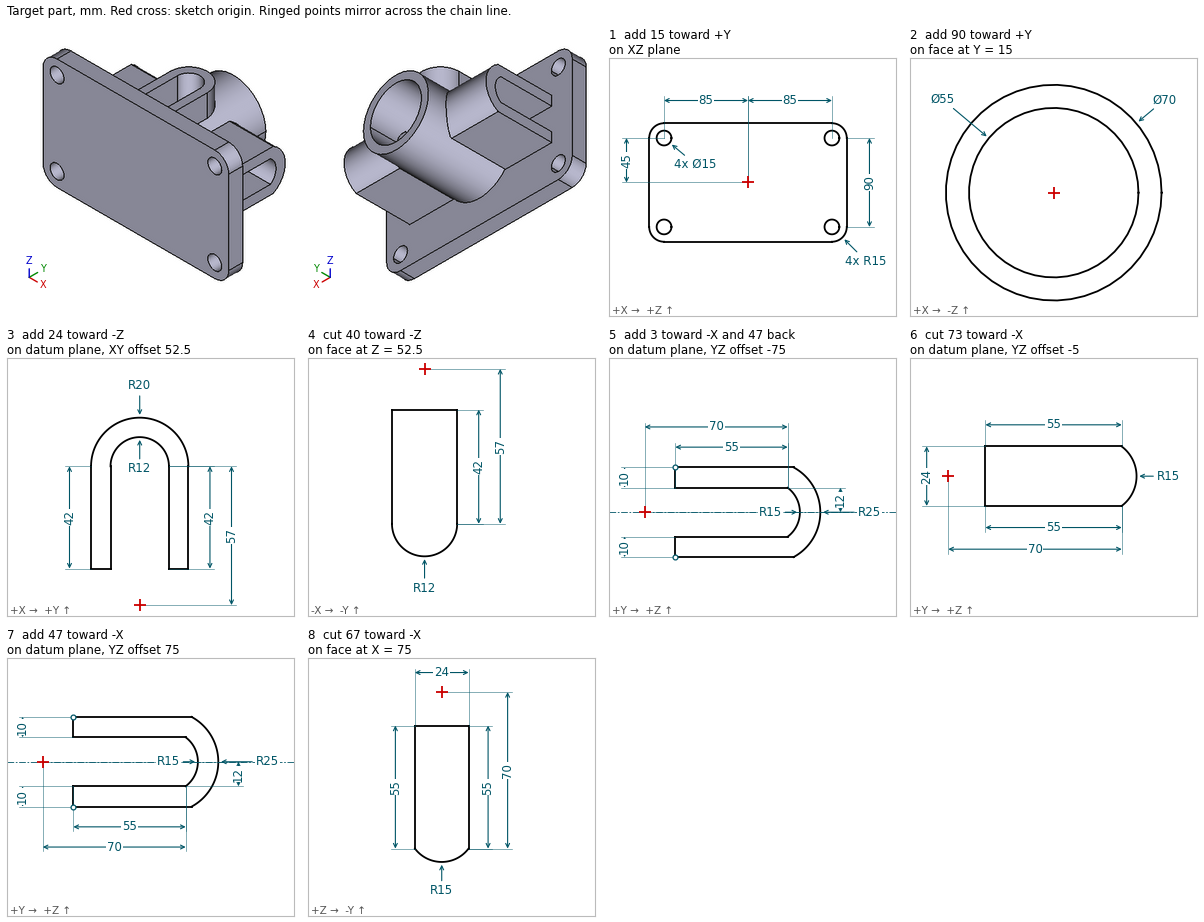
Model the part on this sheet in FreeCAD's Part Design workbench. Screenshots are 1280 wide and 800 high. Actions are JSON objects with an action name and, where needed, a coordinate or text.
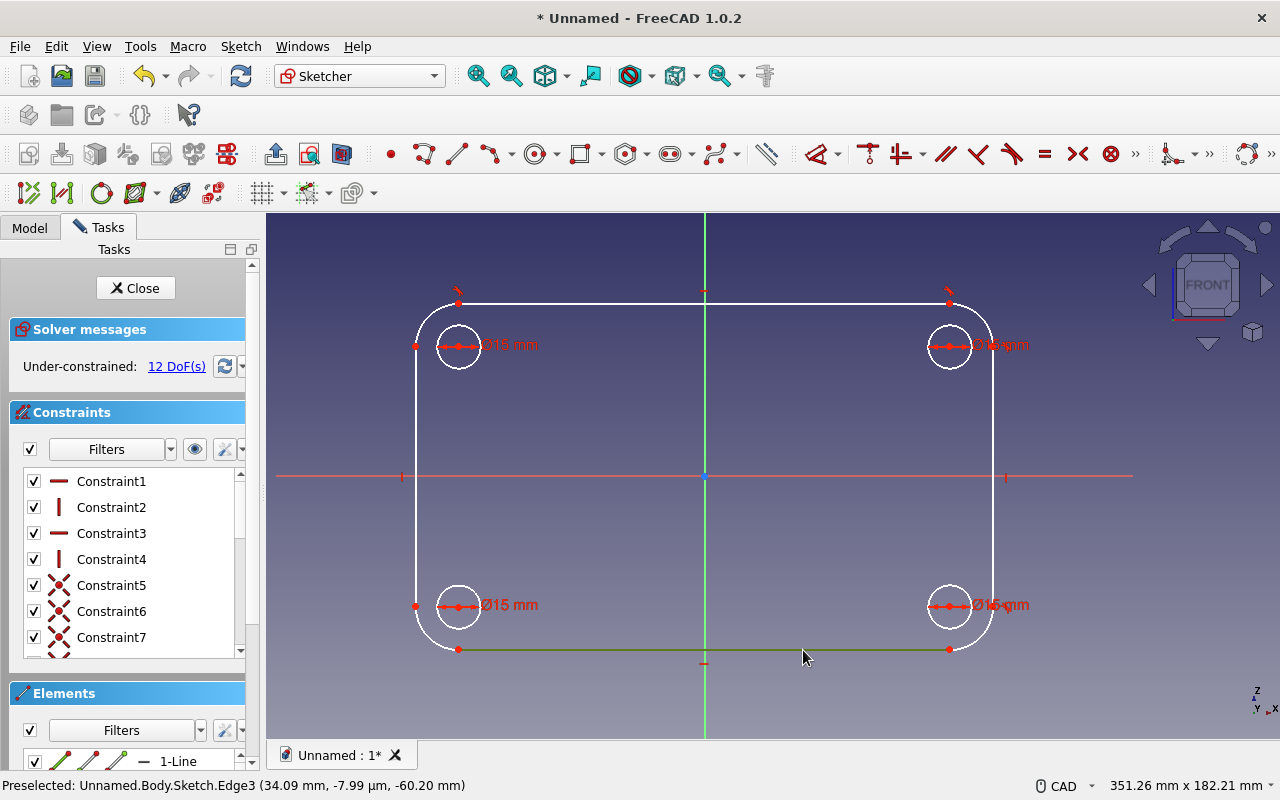
{"action": "left_click", "coordinate": [970, 645]}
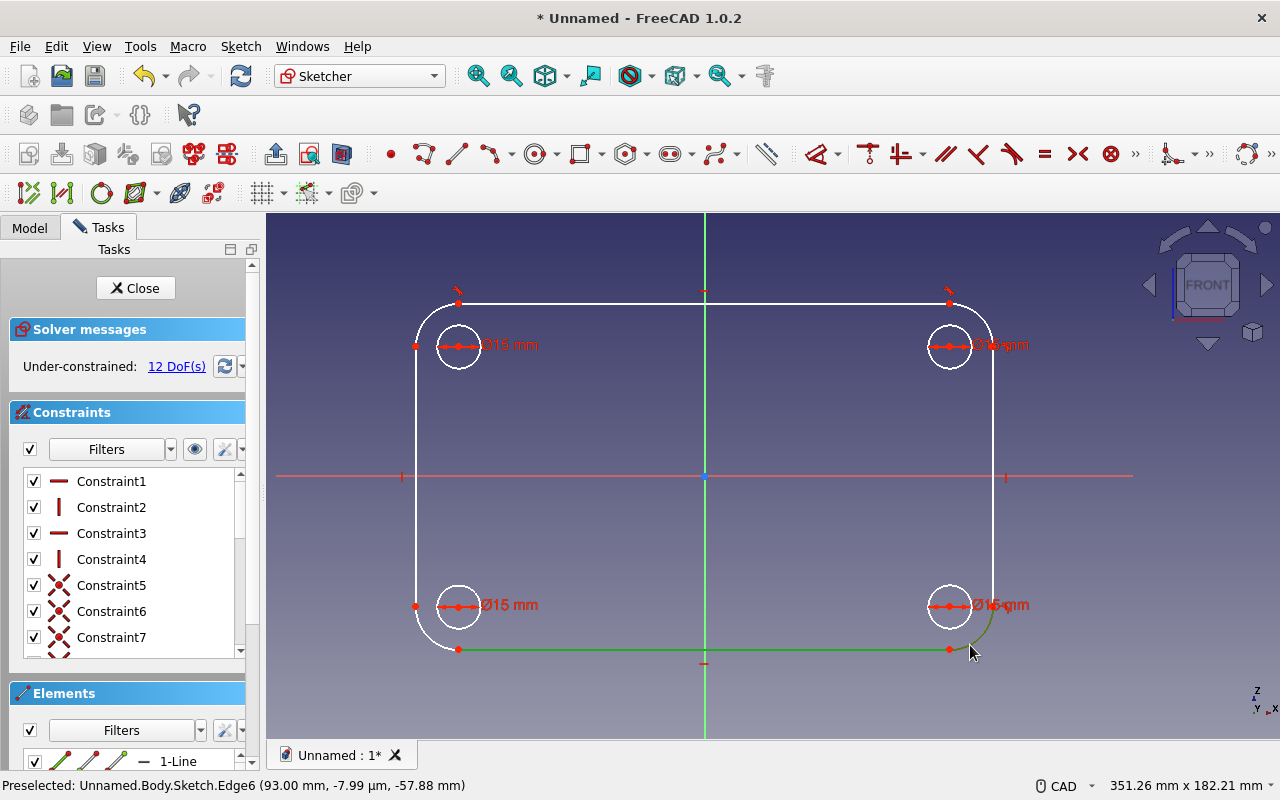
{"action": "key", "text": "t"}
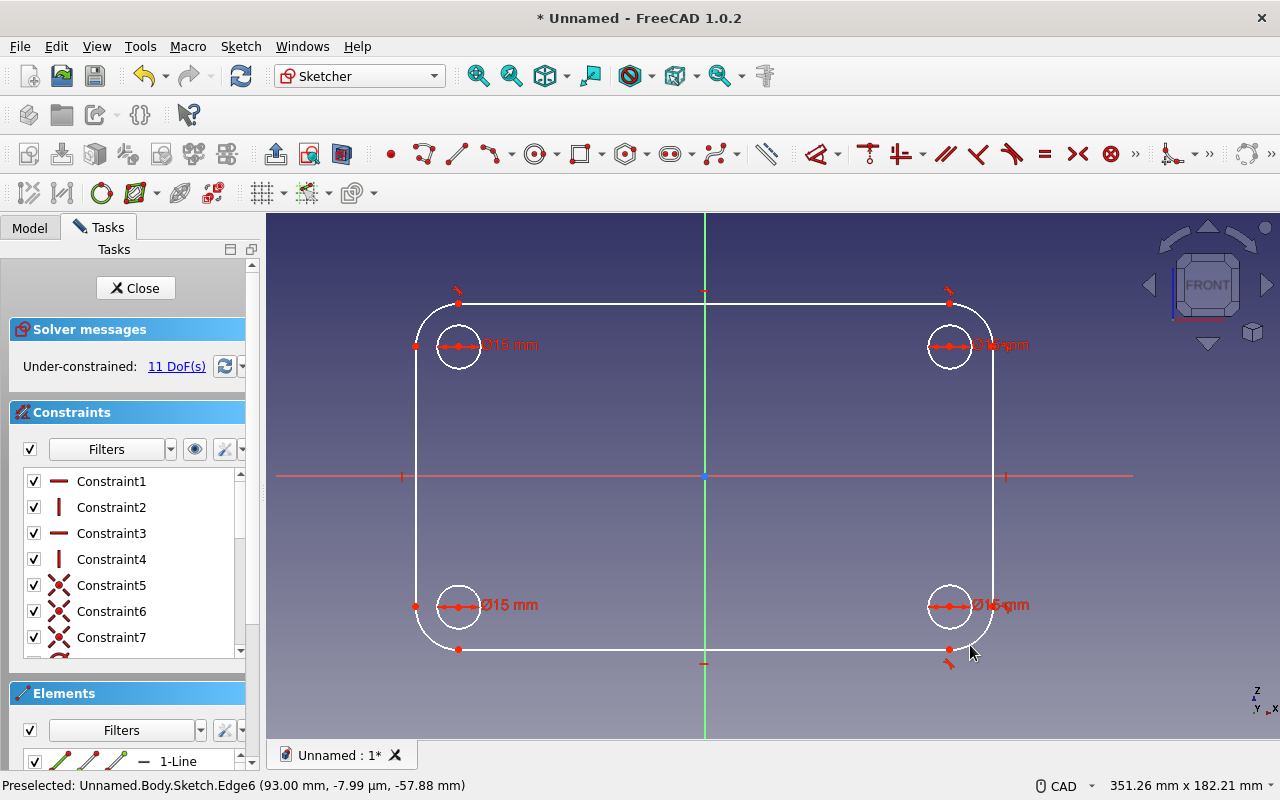
{"action": "left_click", "coordinate": [803, 650]}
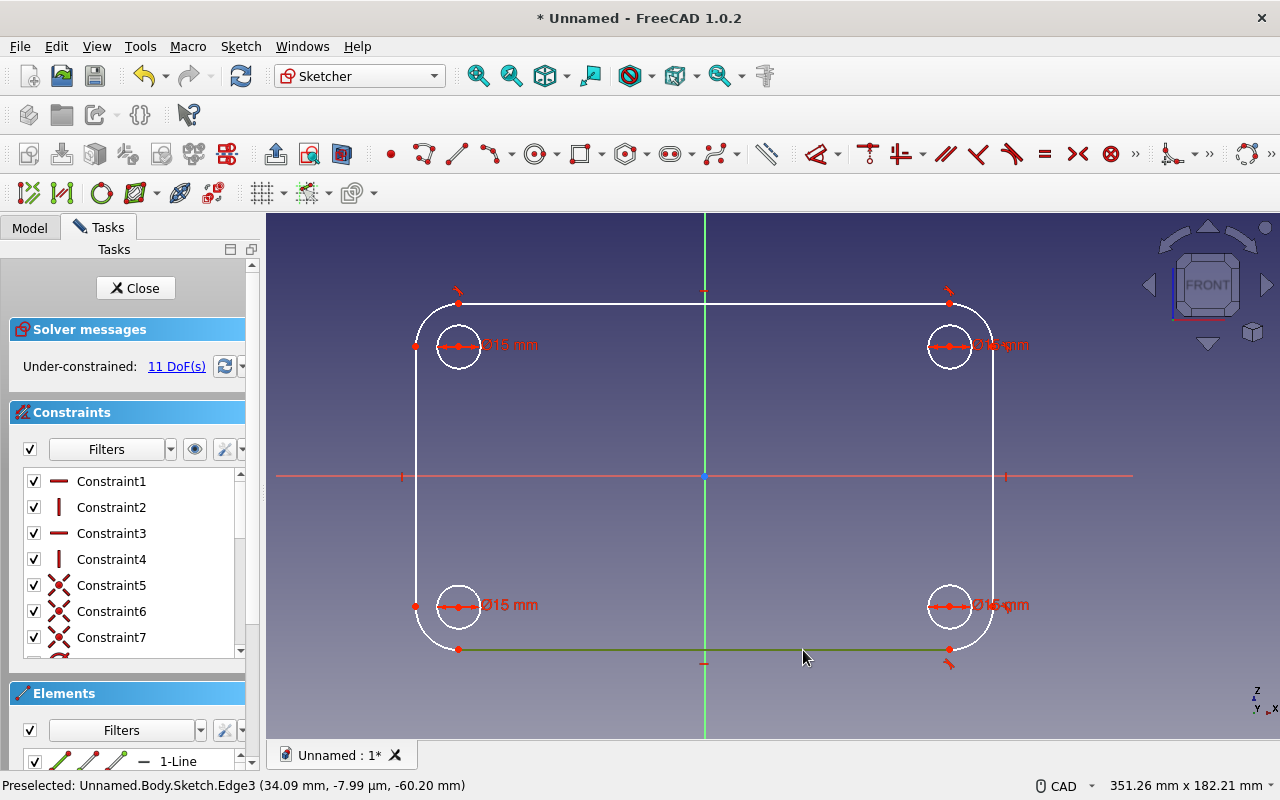
{"action": "left_click", "coordinate": [421, 627]}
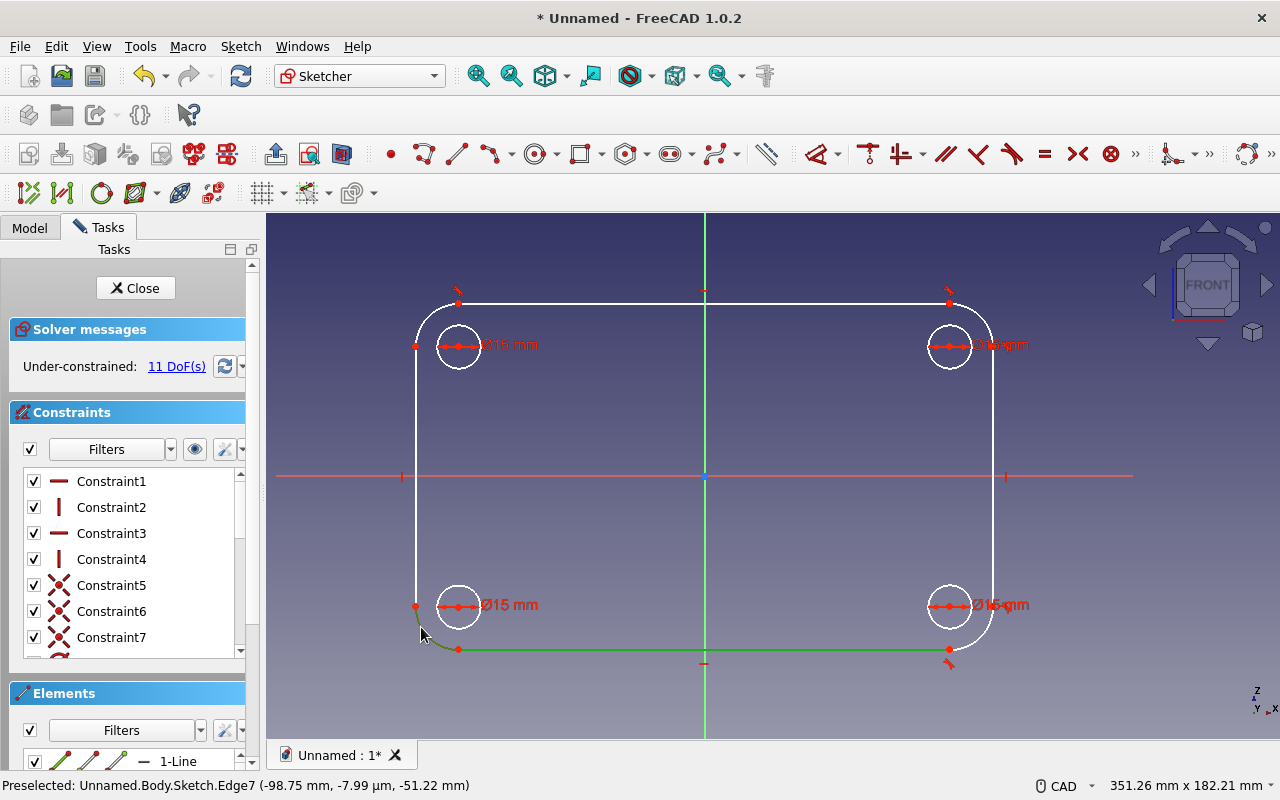
{"action": "key", "text": "t"}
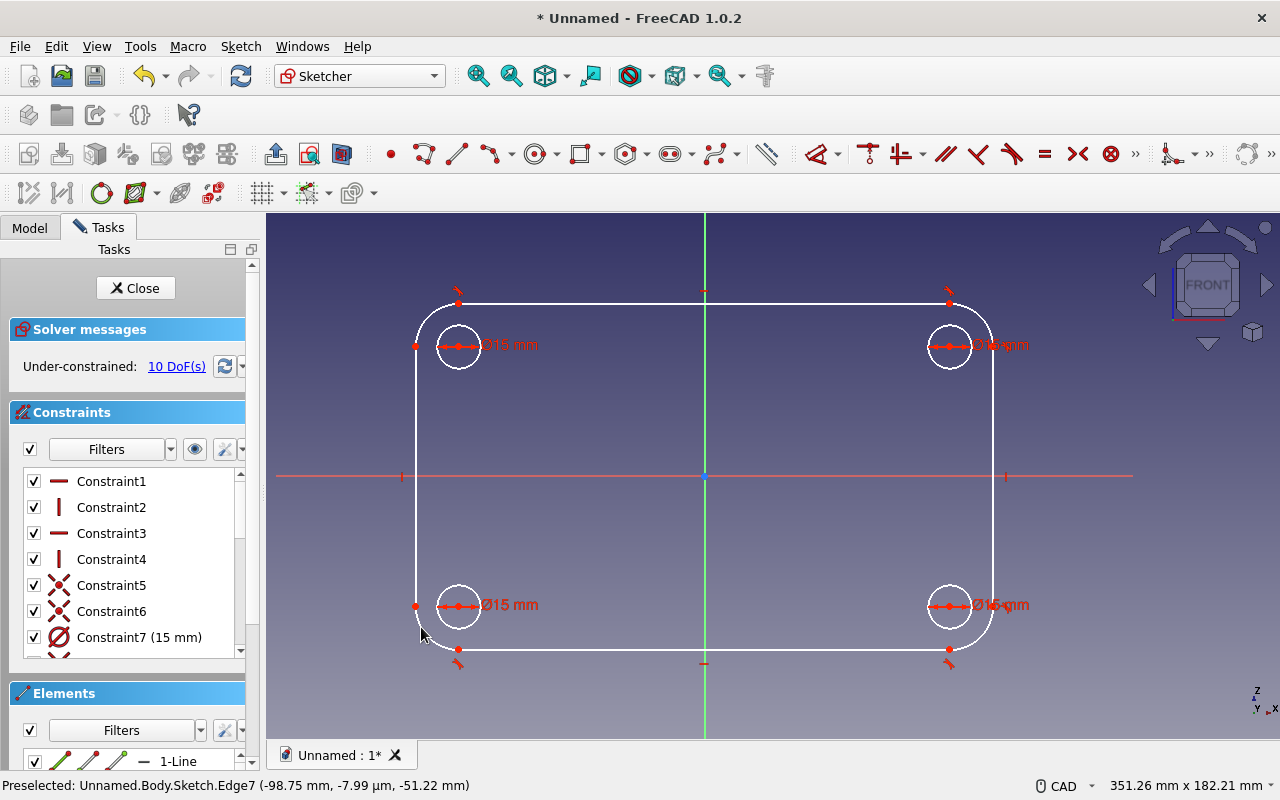
{"action": "left_click", "coordinate": [416, 529]}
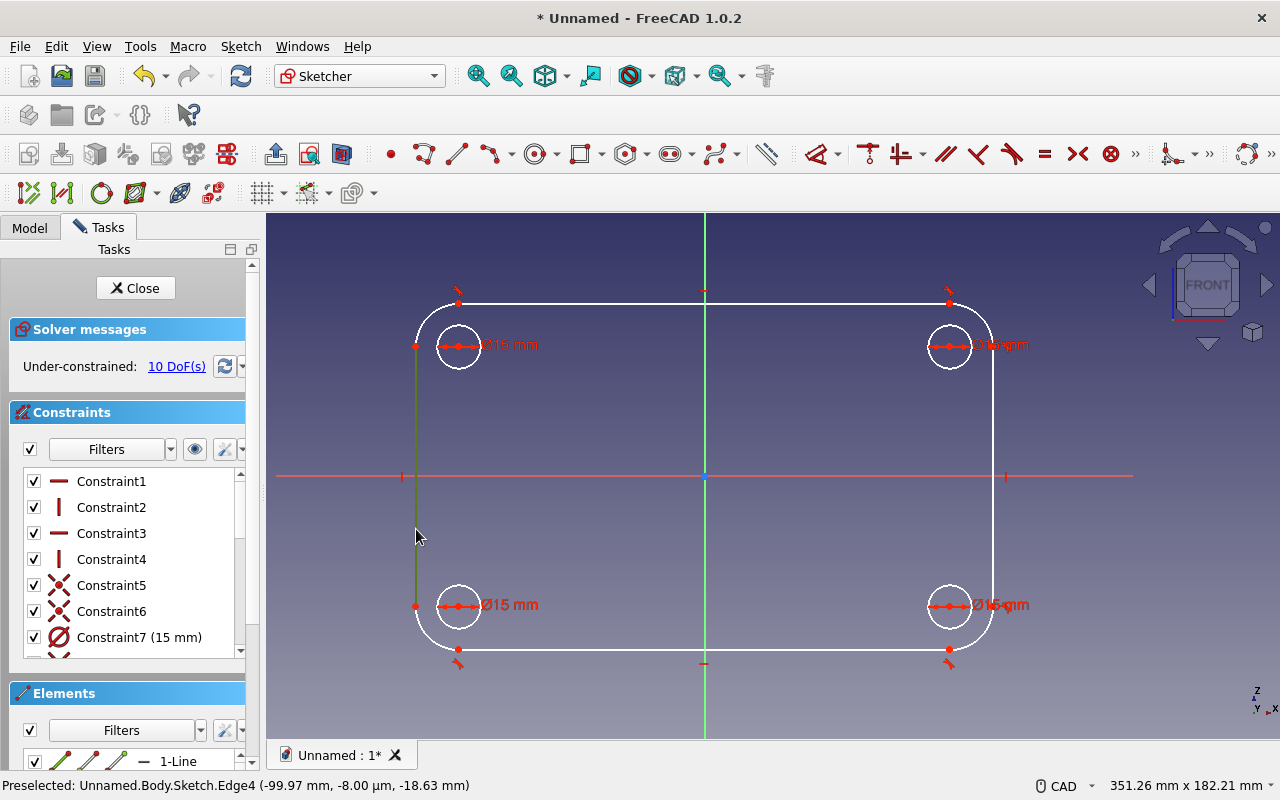
{"action": "left_click", "coordinate": [421, 627]}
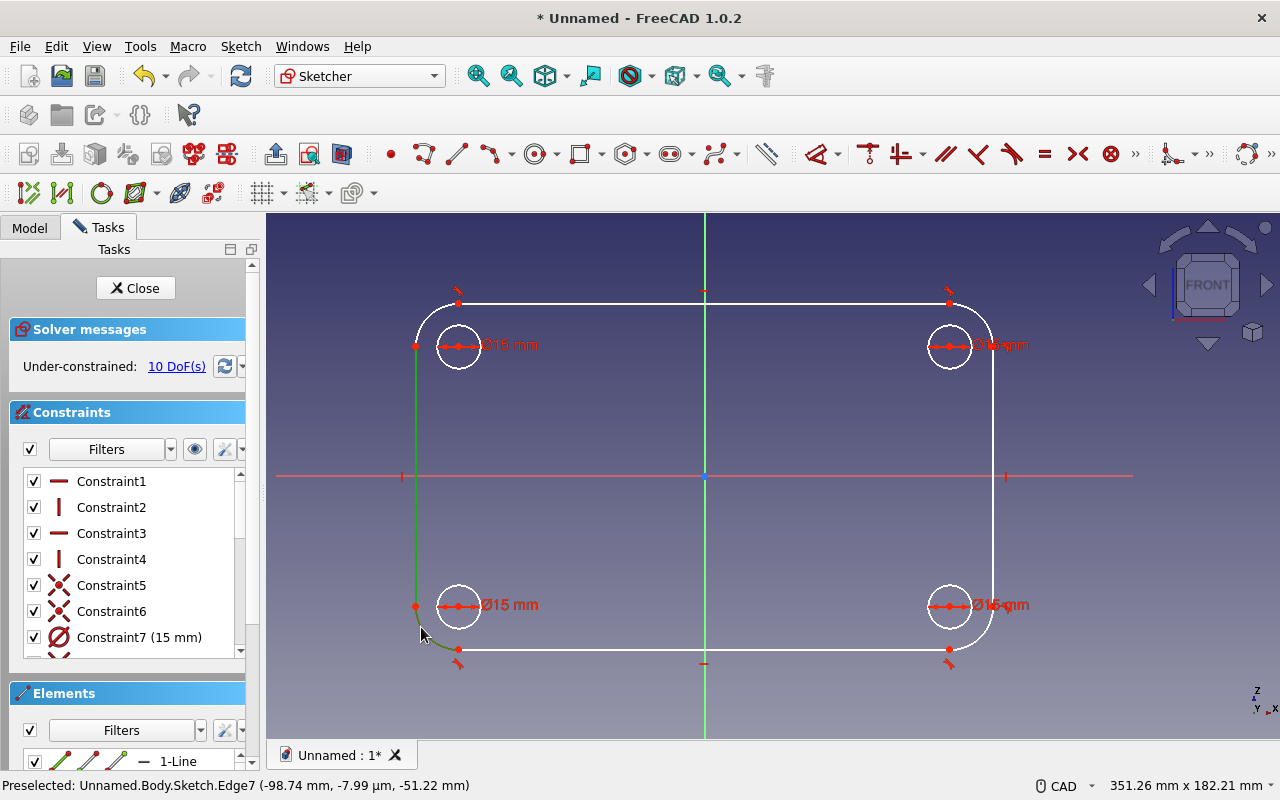
{"action": "key", "text": "t"}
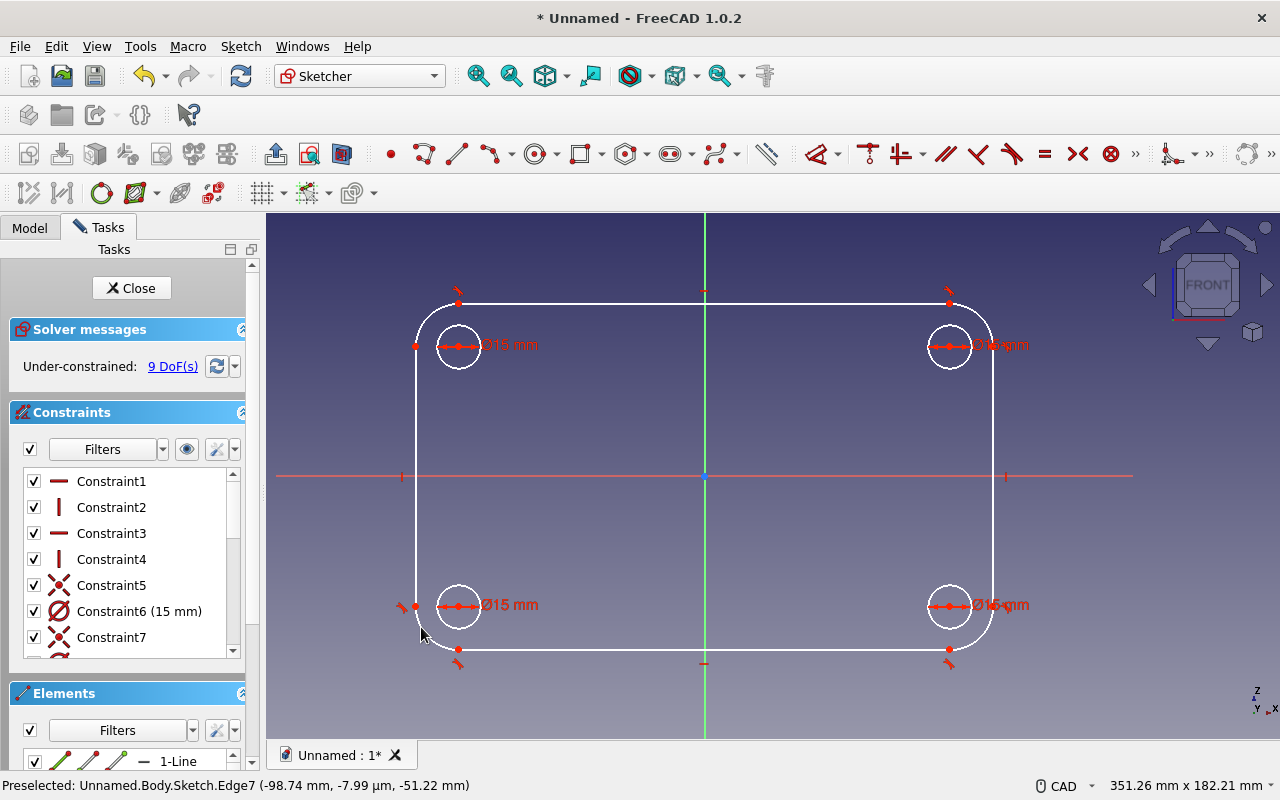
{"action": "left_click", "coordinate": [416, 529]}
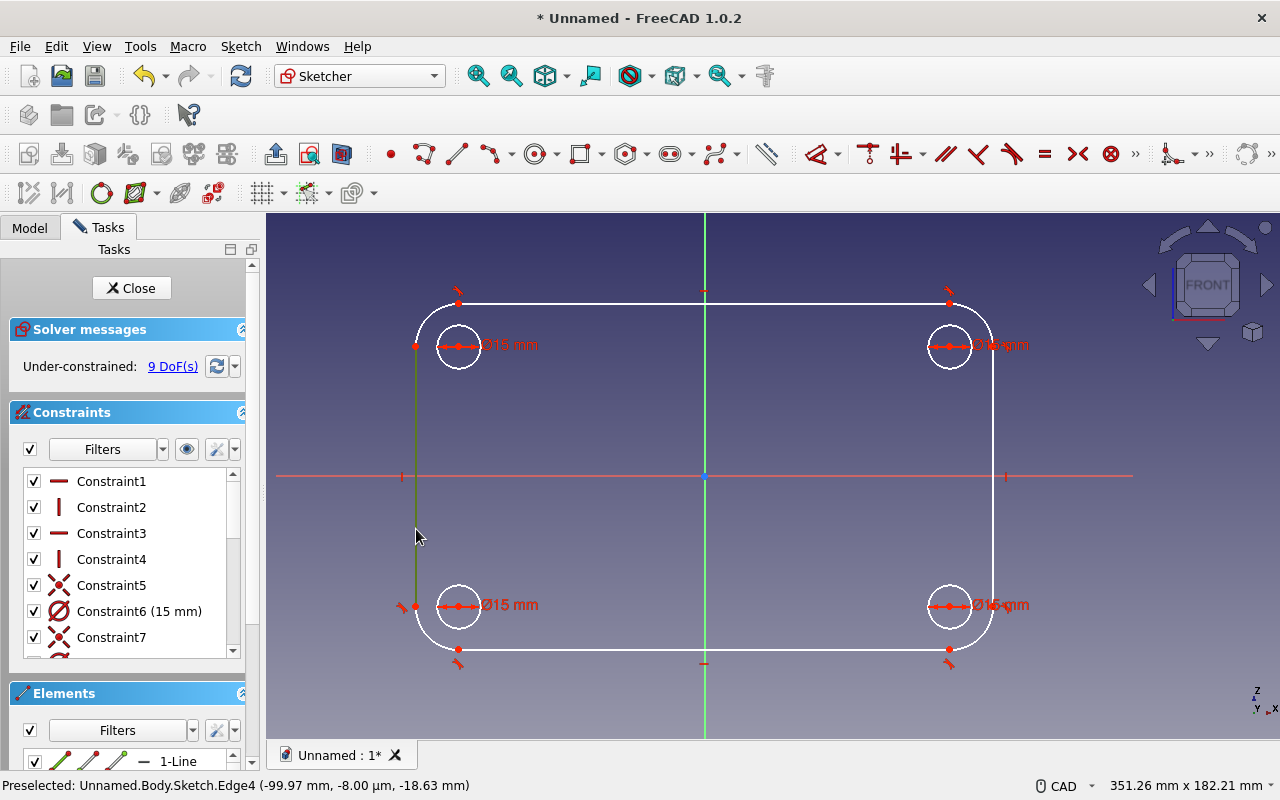
{"action": "left_click", "coordinate": [439, 309]}